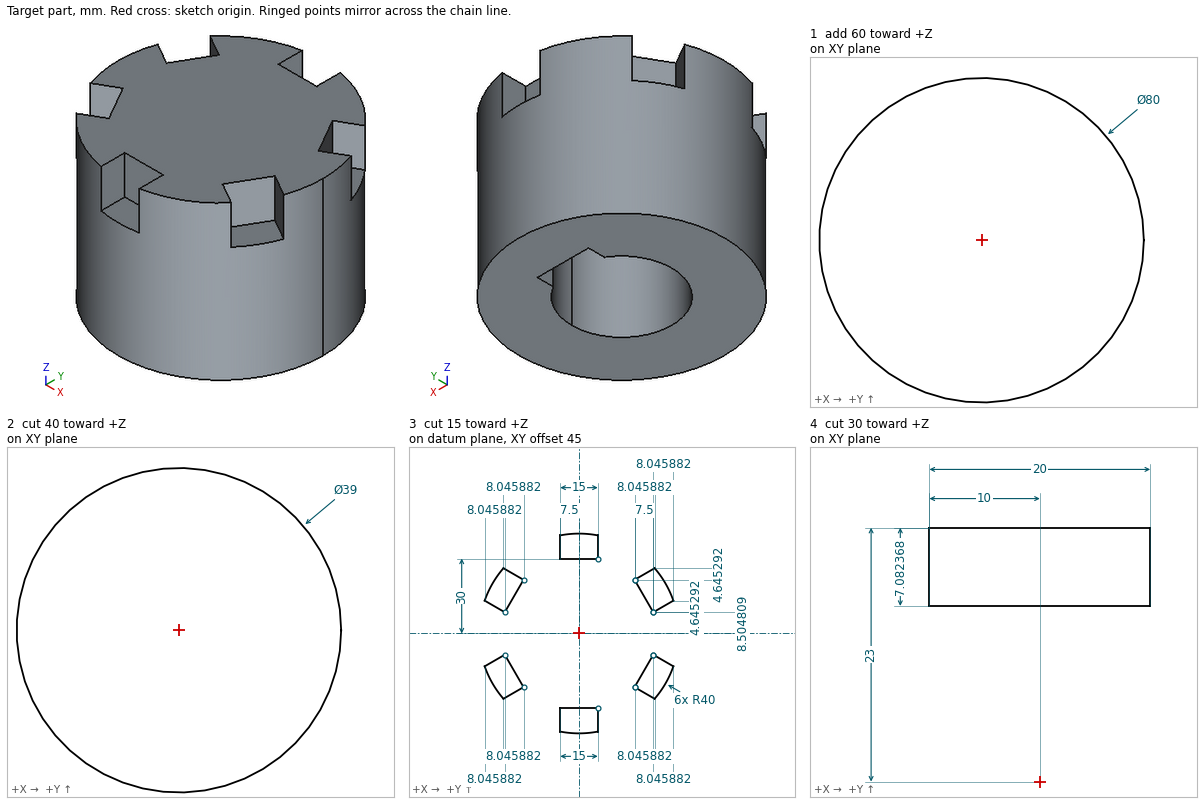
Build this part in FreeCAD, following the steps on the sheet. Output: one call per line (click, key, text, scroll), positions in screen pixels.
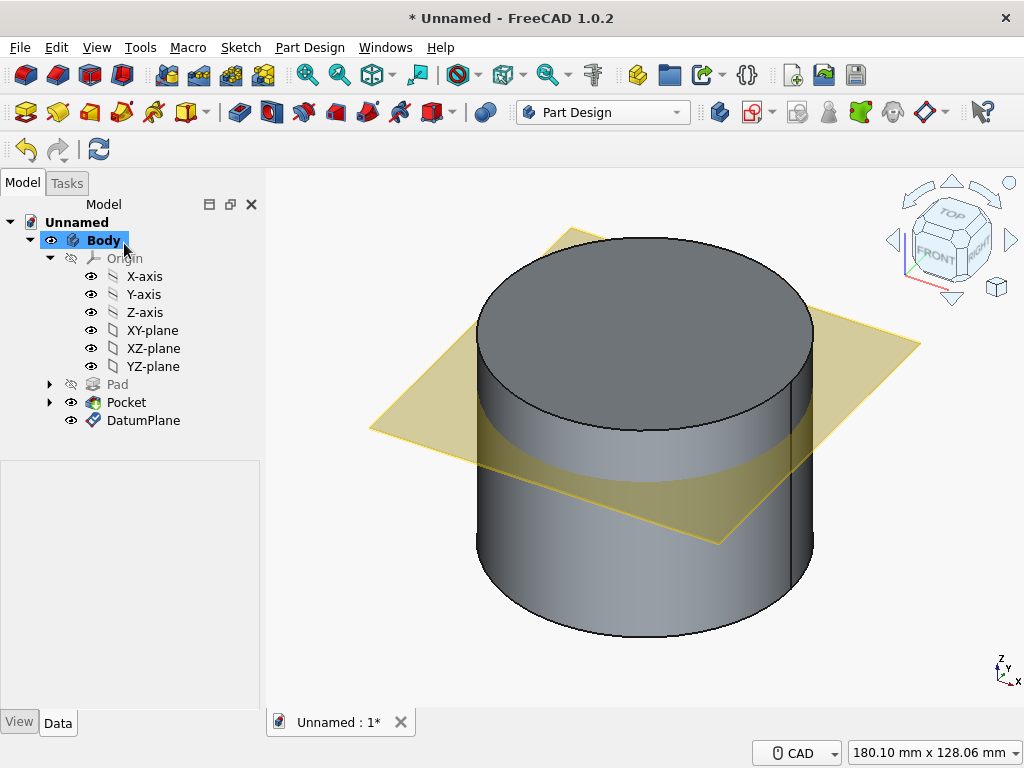
click(116, 420)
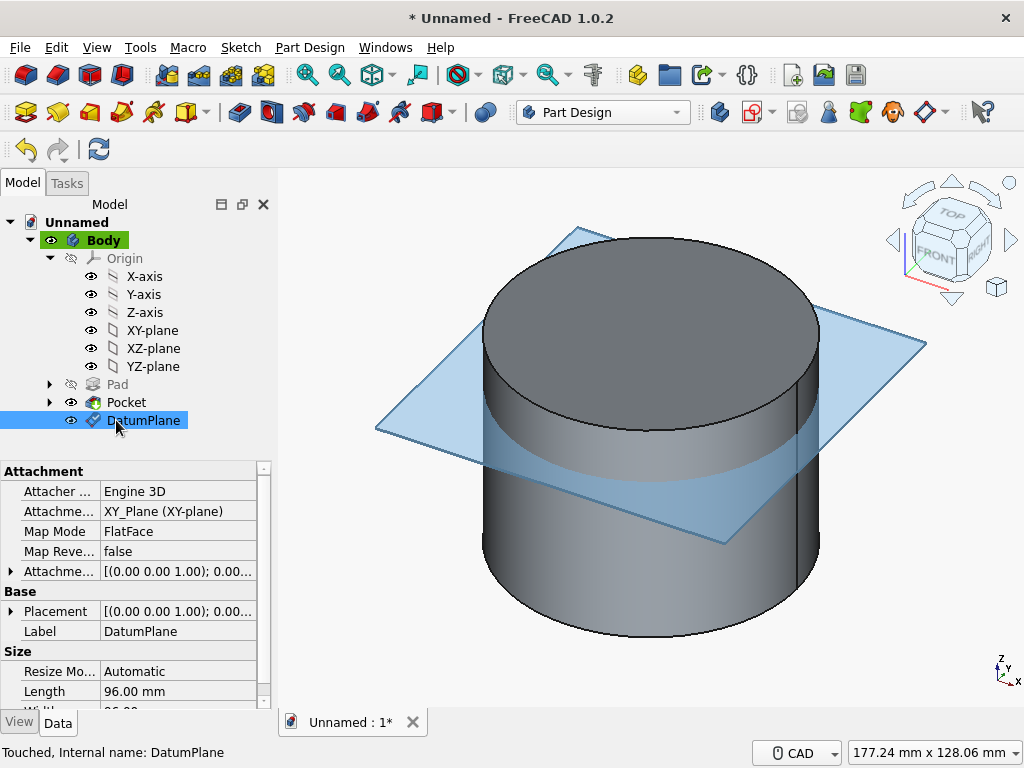
click(752, 112)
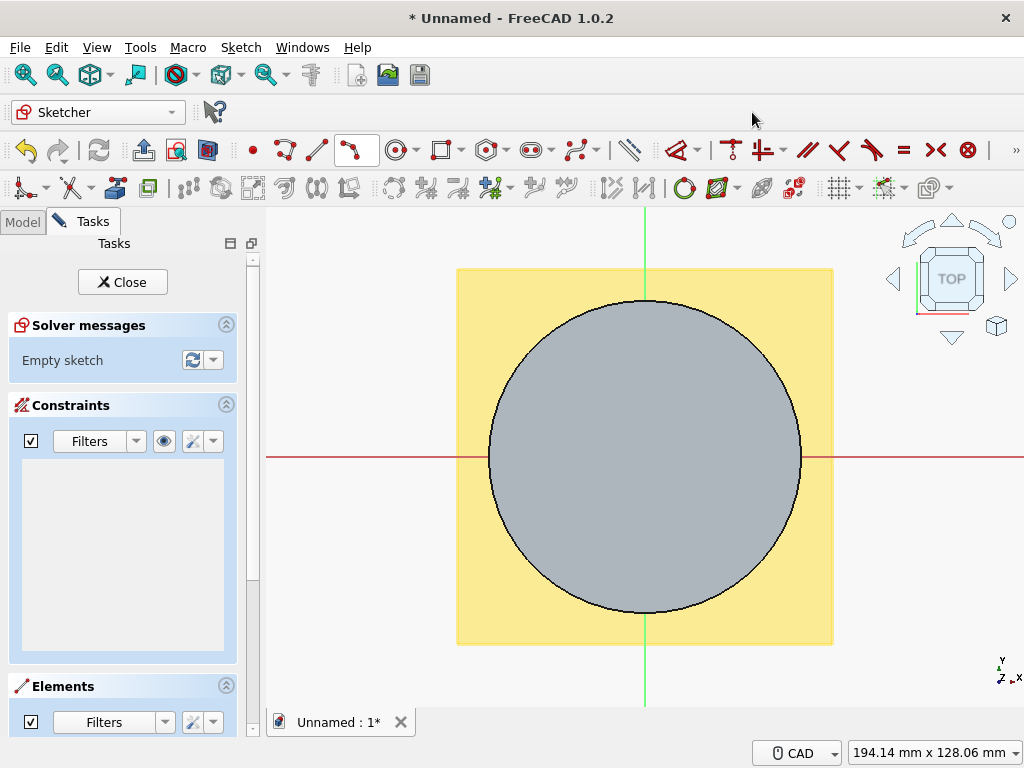
key(q)
key(s)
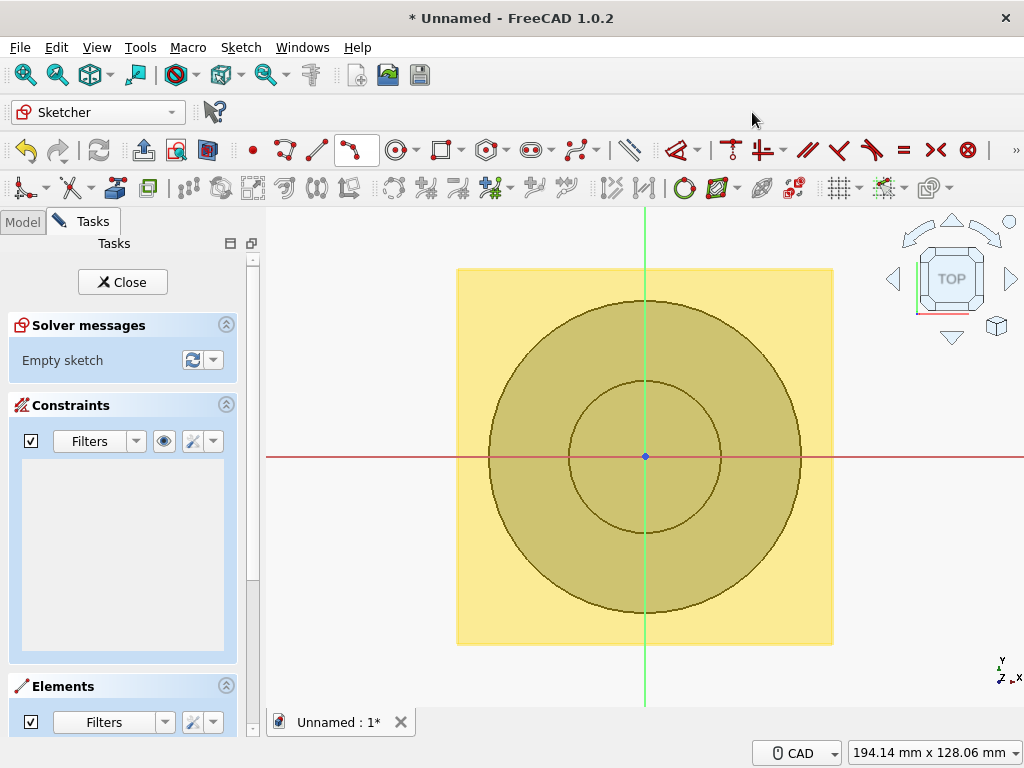
click(286, 150)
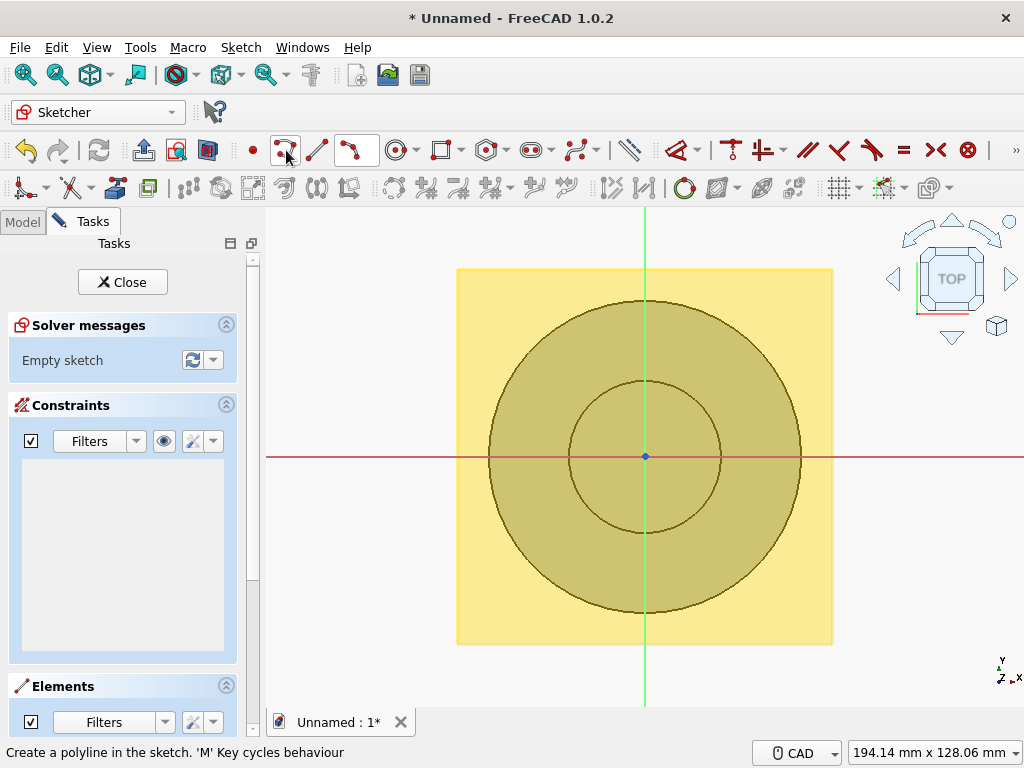
click(763, 355)
click(732, 373)
click(761, 424)
click(792, 406)
right_click(792, 406)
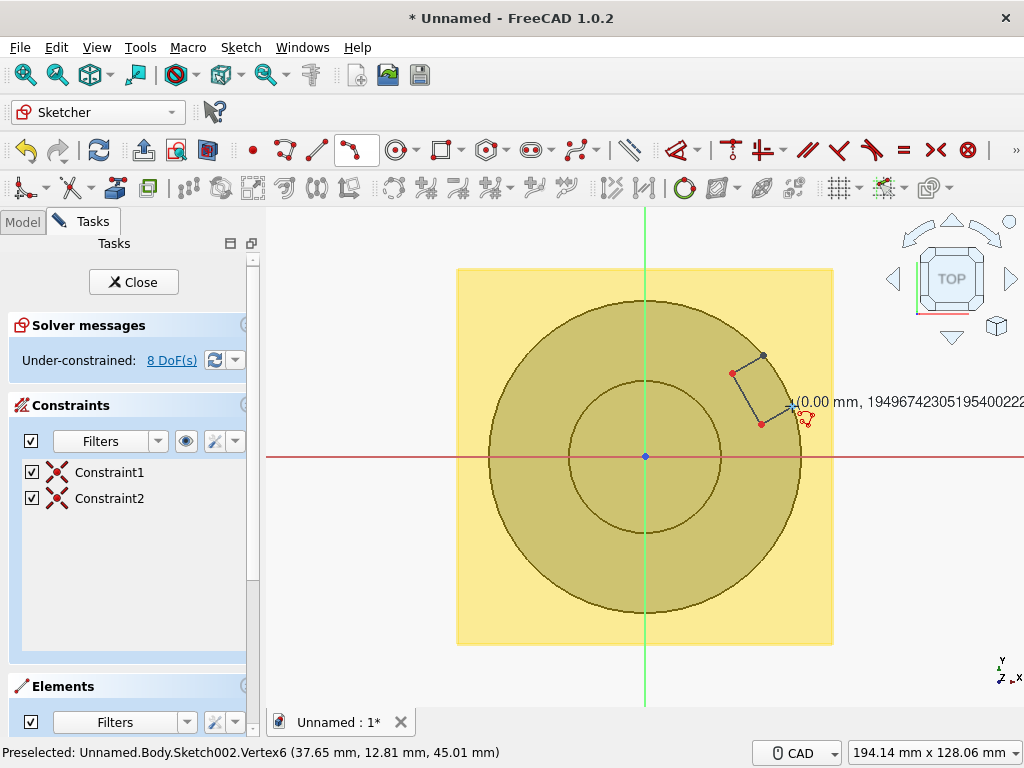
click(350, 150)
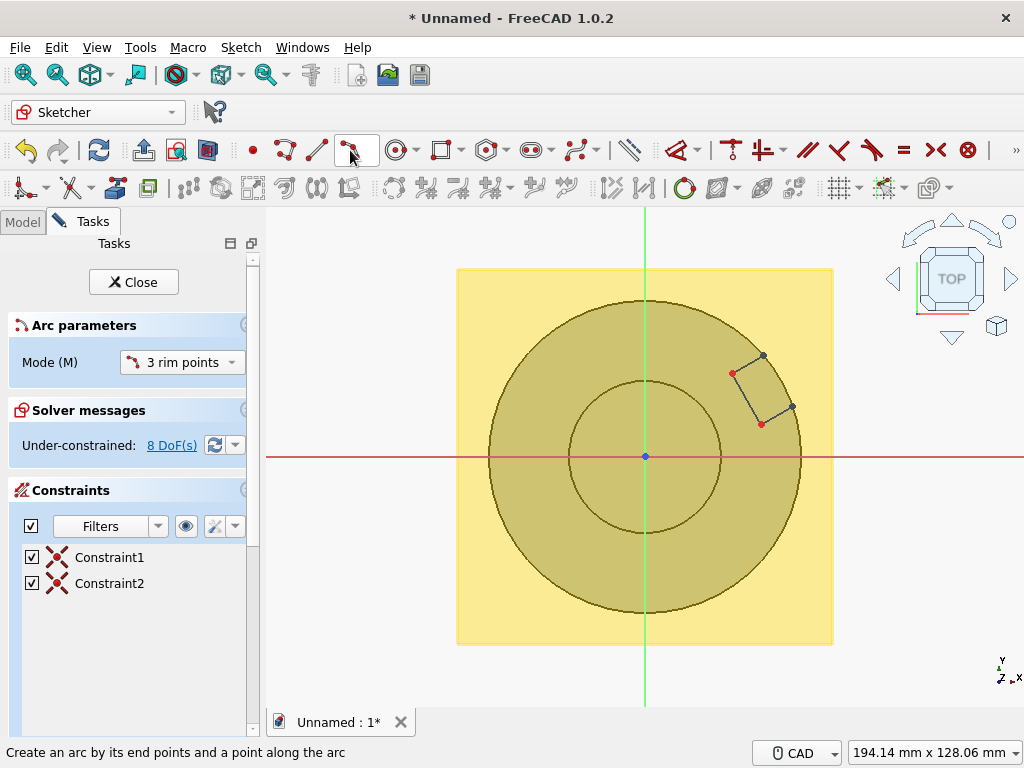
click(792, 407)
click(763, 356)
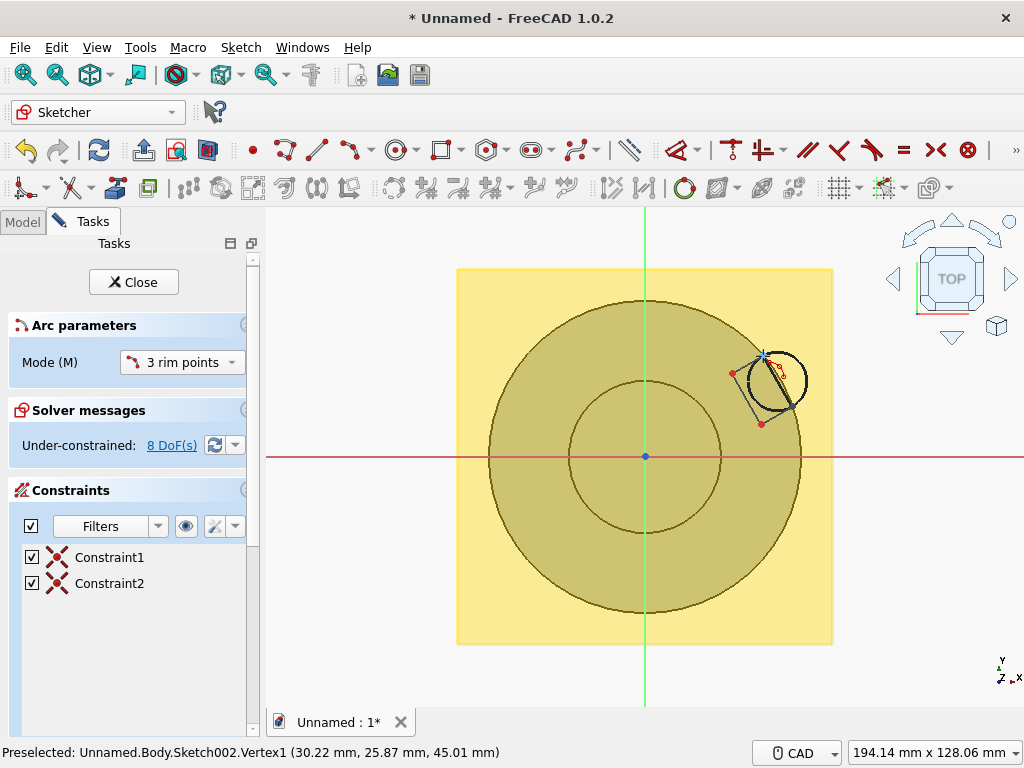
scroll(780, 379, up, 9)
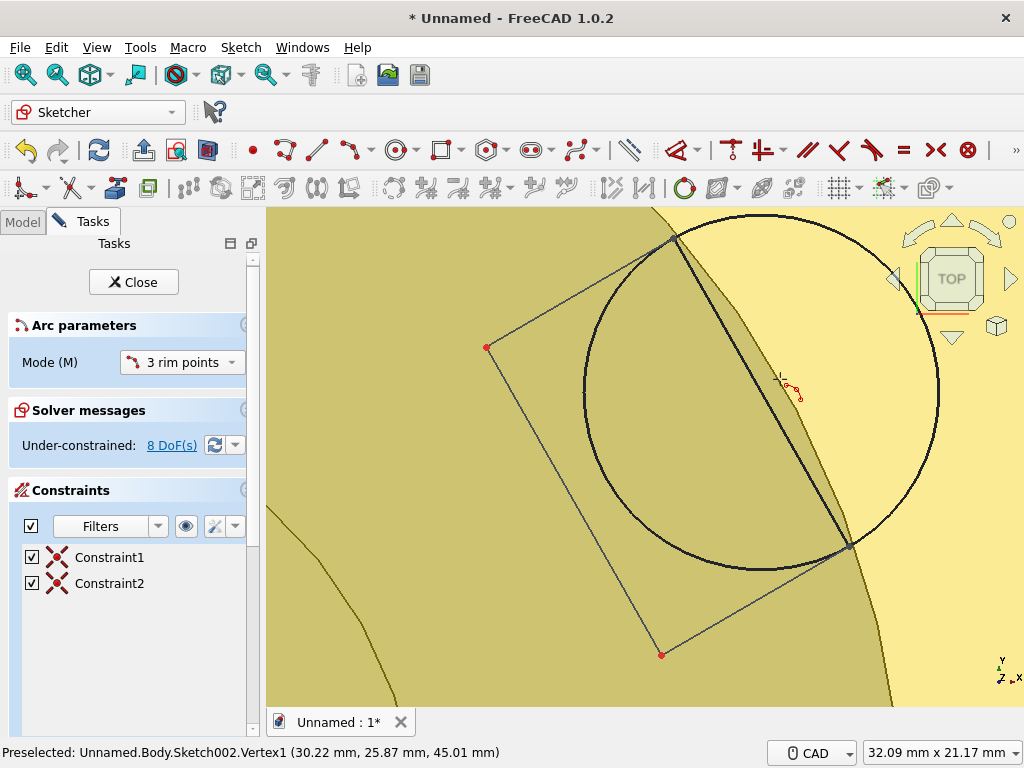
click(778, 377)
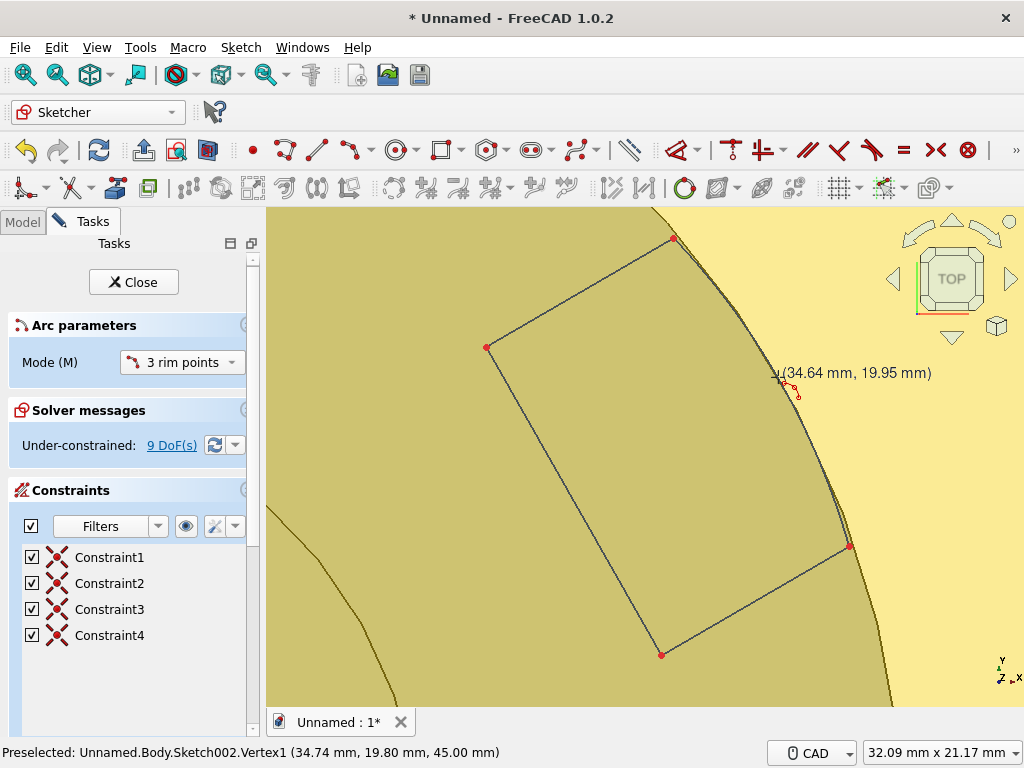
click(286, 150)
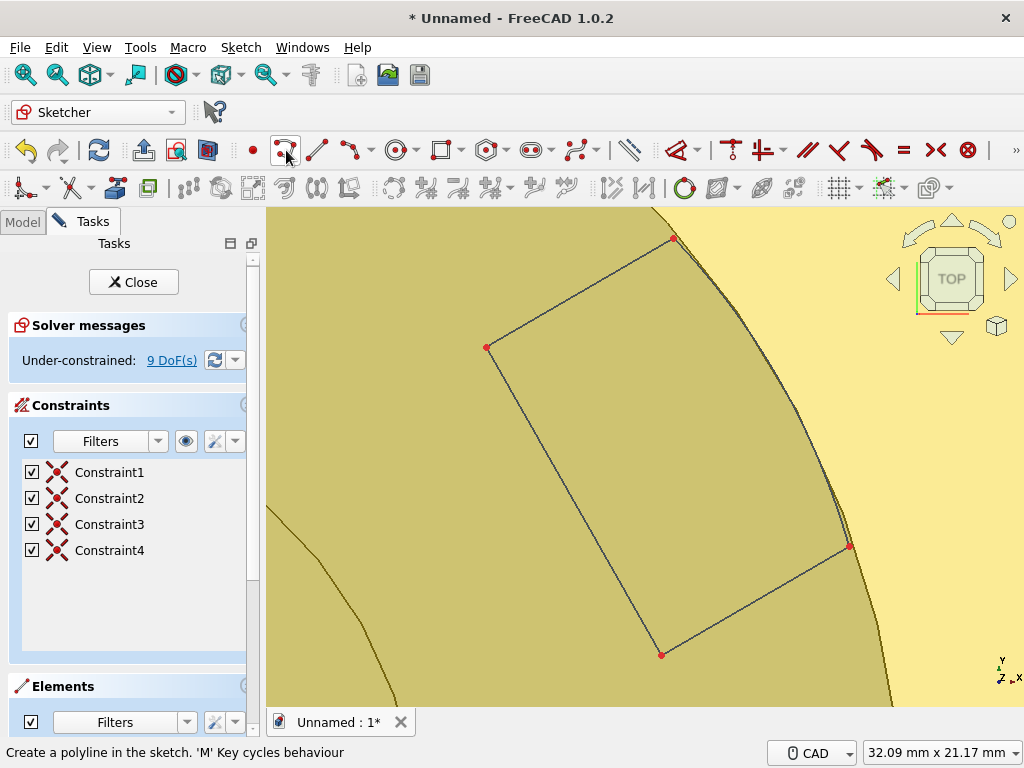
scroll(699, 379, down, 9)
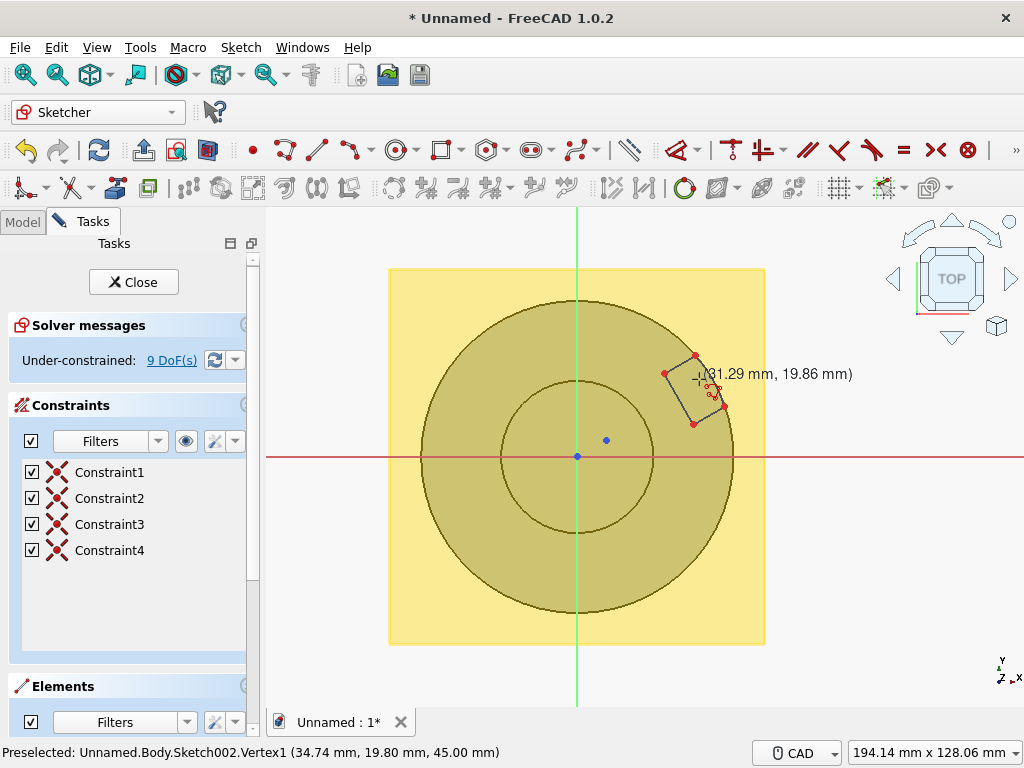
click(548, 304)
click(548, 340)
click(607, 340)
click(607, 304)
right_click(607, 304)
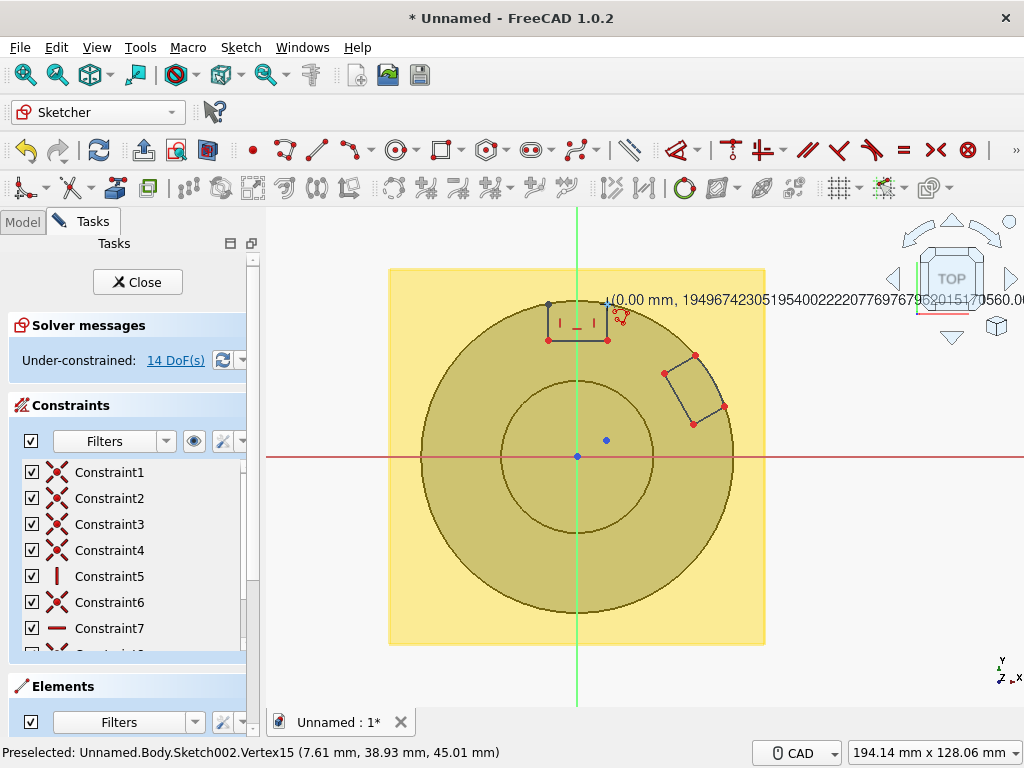
key(g)
key(3)
key(a)